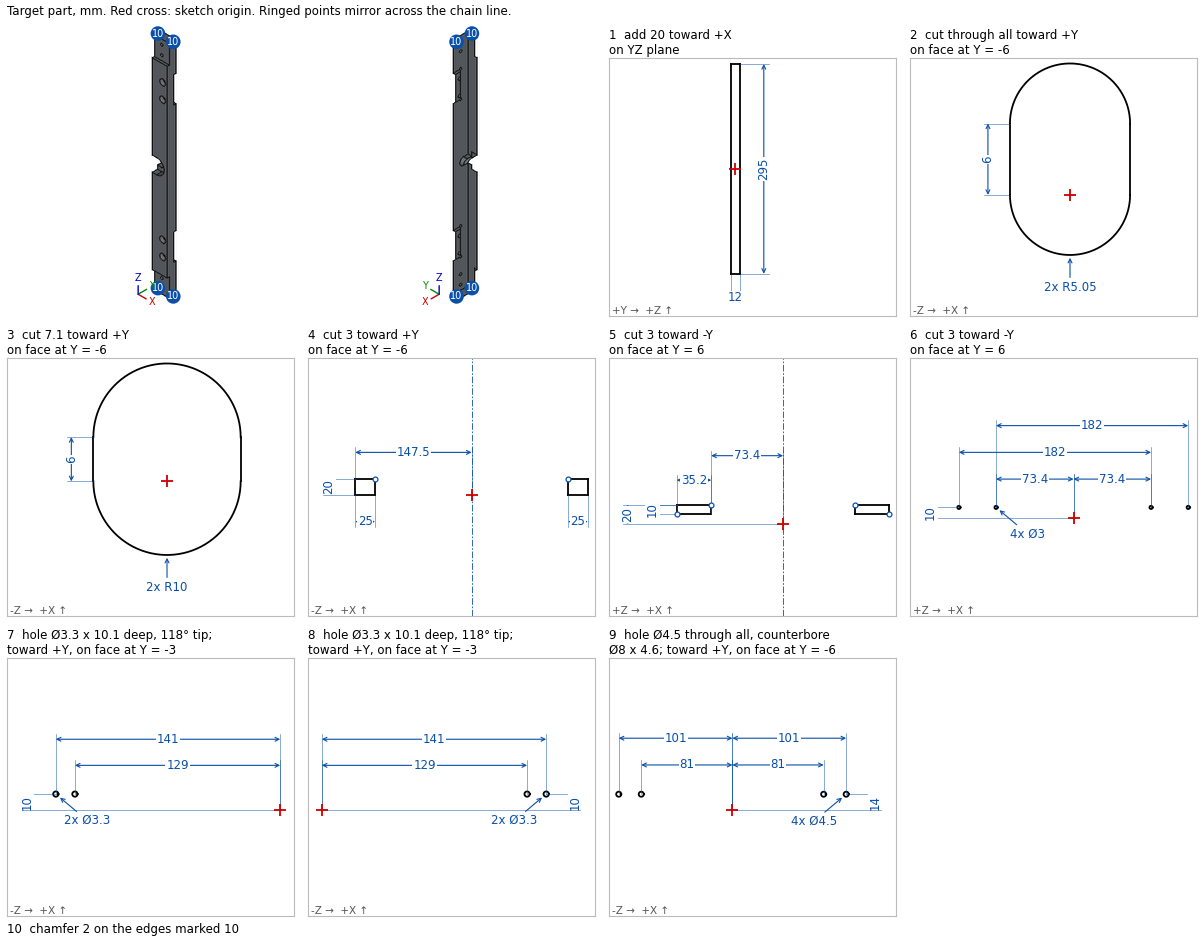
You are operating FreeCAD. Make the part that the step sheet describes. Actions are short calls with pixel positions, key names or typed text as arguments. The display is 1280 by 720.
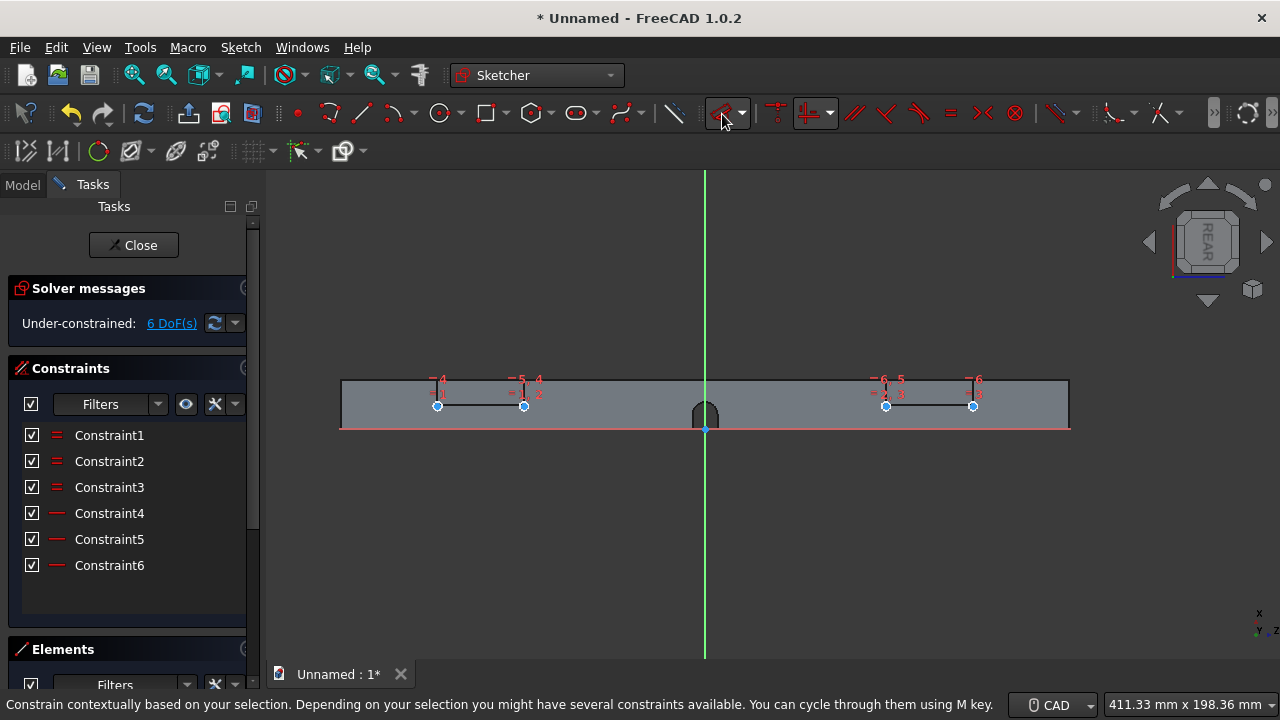
scroll(441, 403, up, 9)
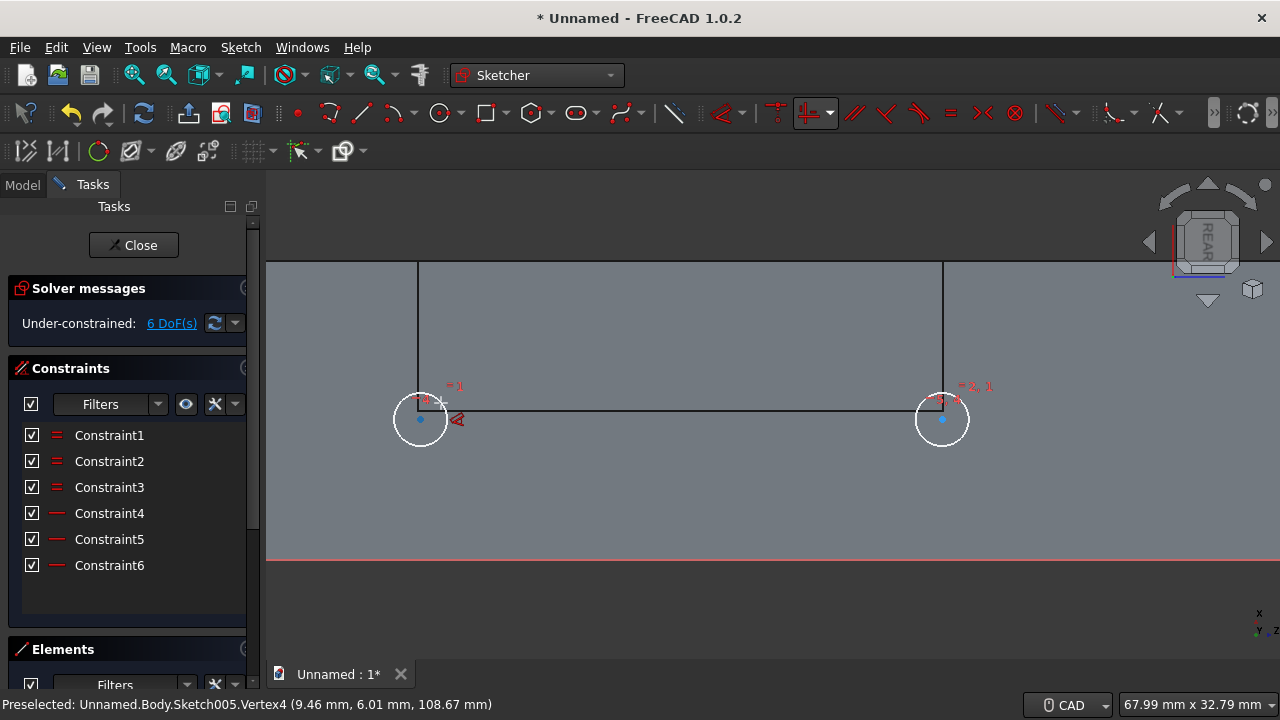
click(439, 401)
click(462, 378)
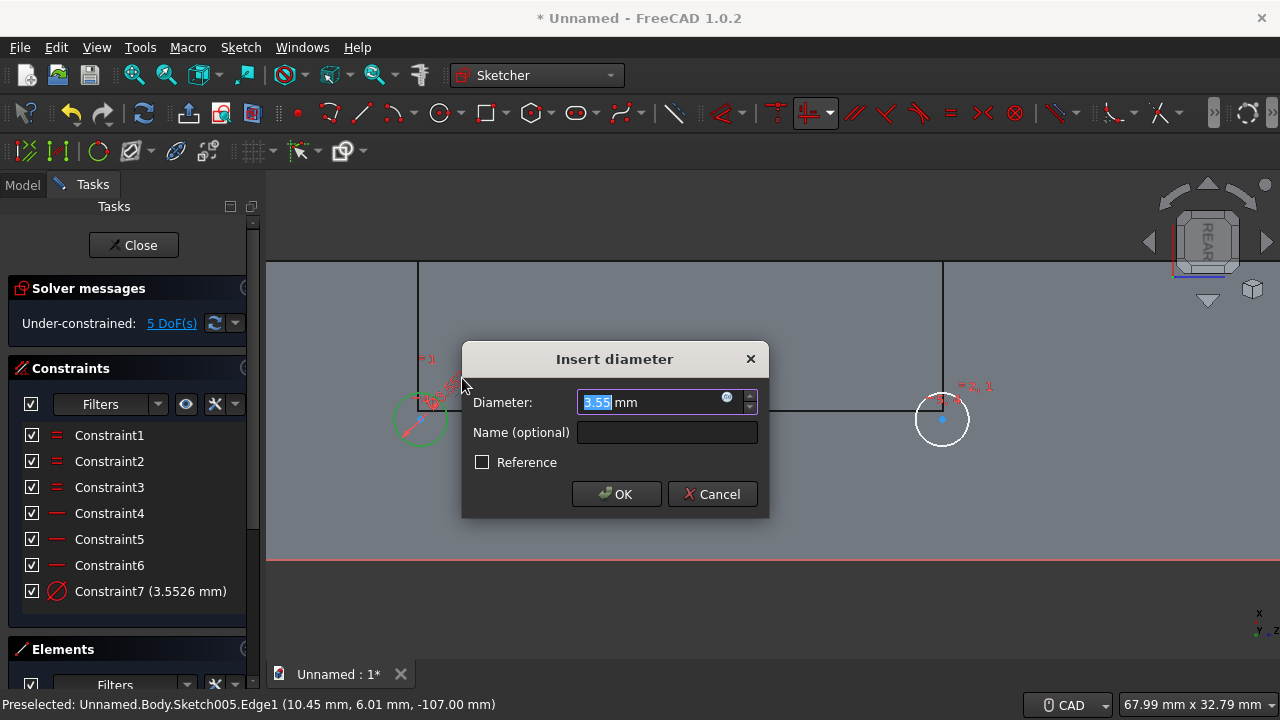
text(3)
key(Return)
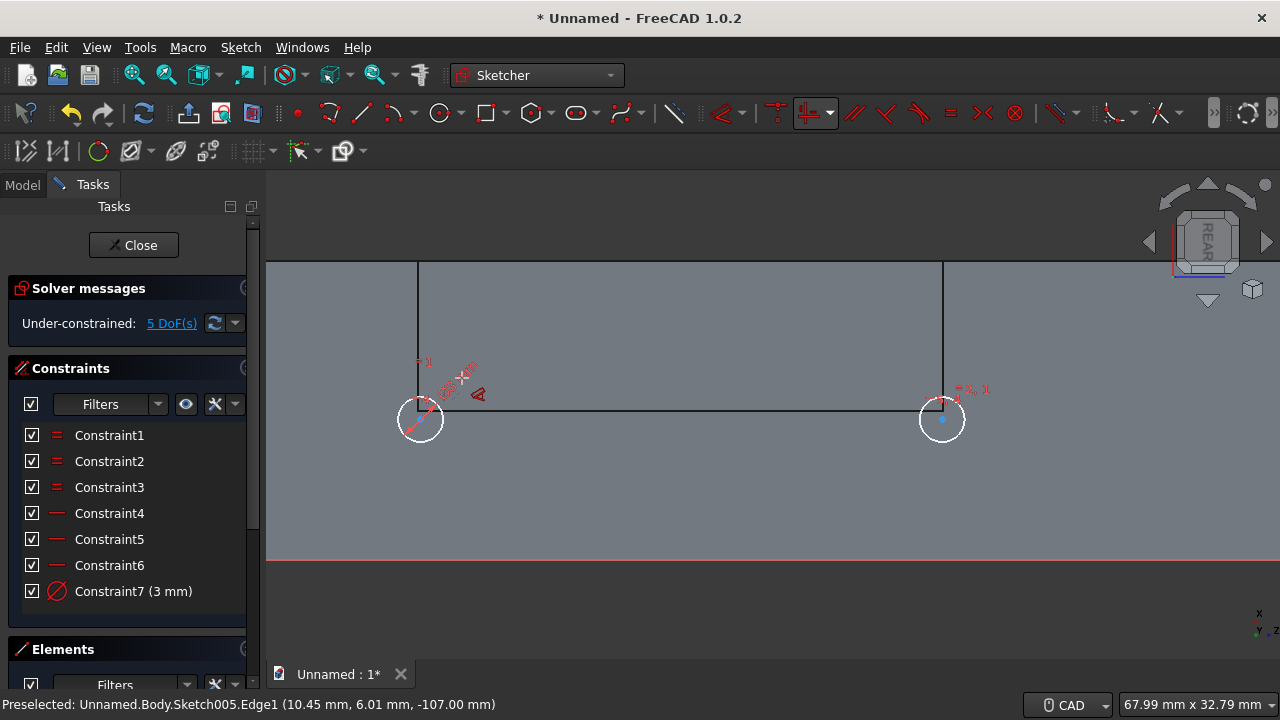
scroll(440, 403, down, 9)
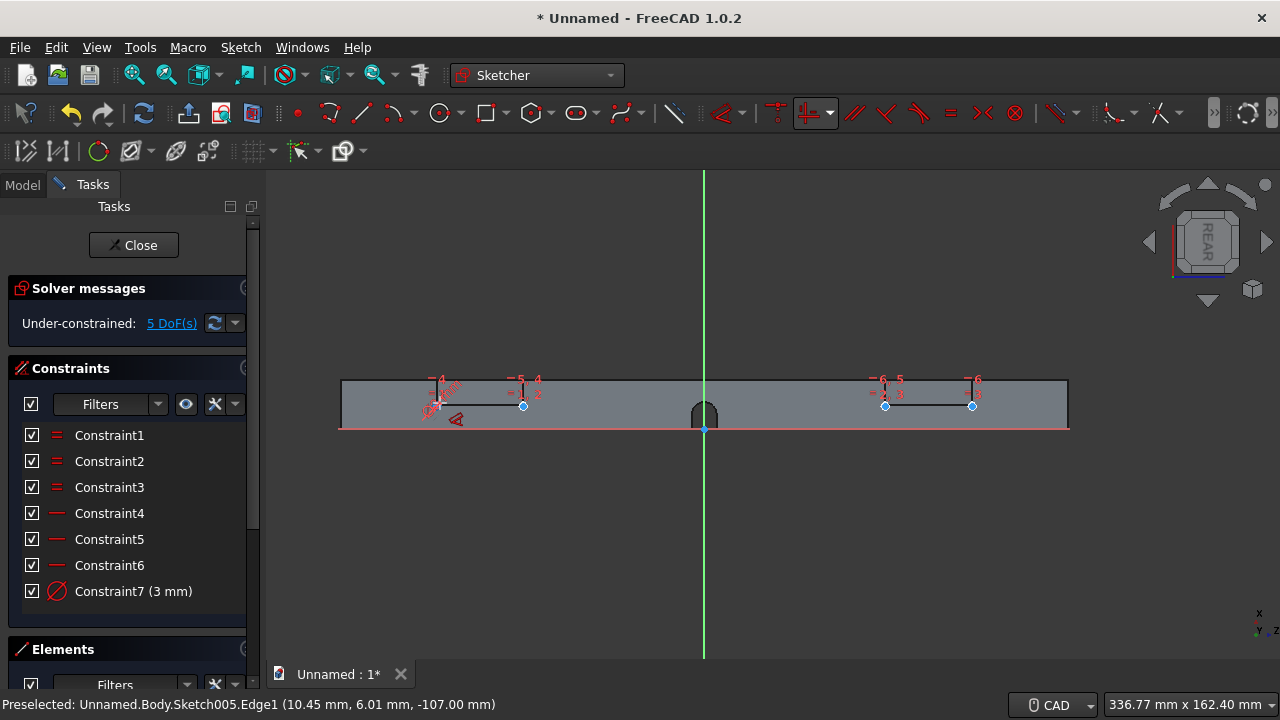
scroll(437, 406, up, 3)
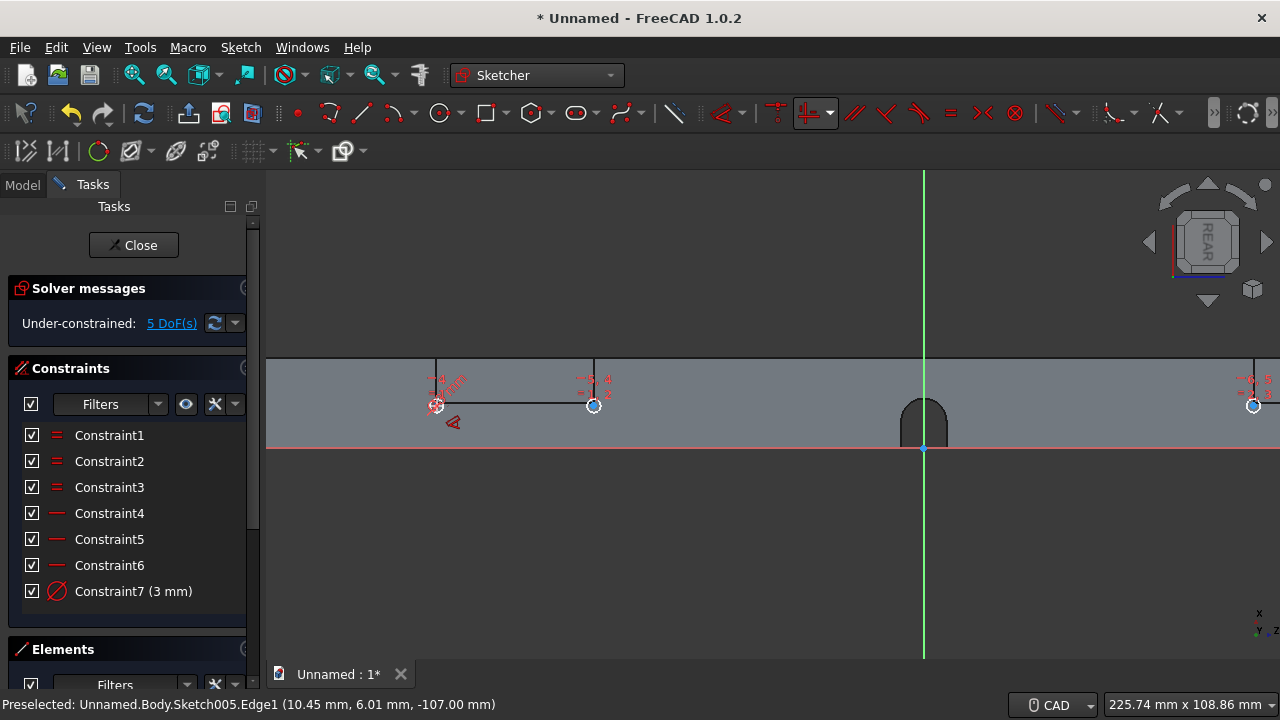
click(437, 406)
click(403, 427)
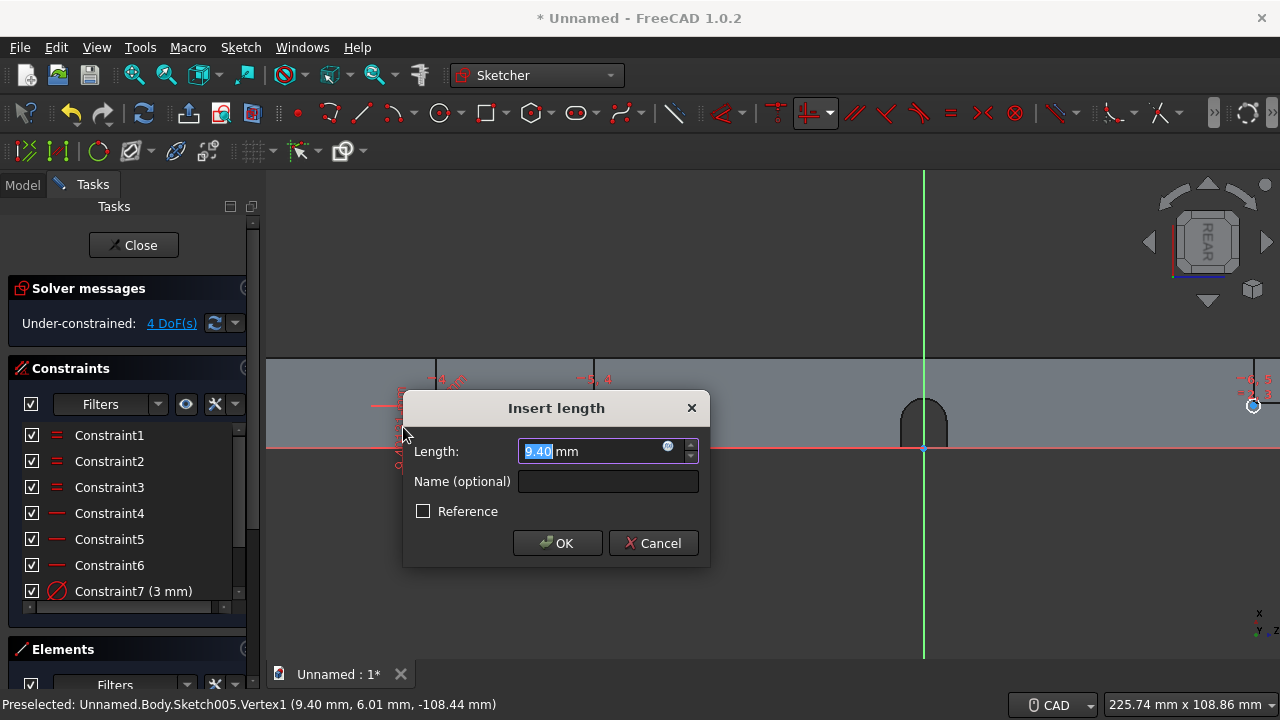
text(10)
key(Return)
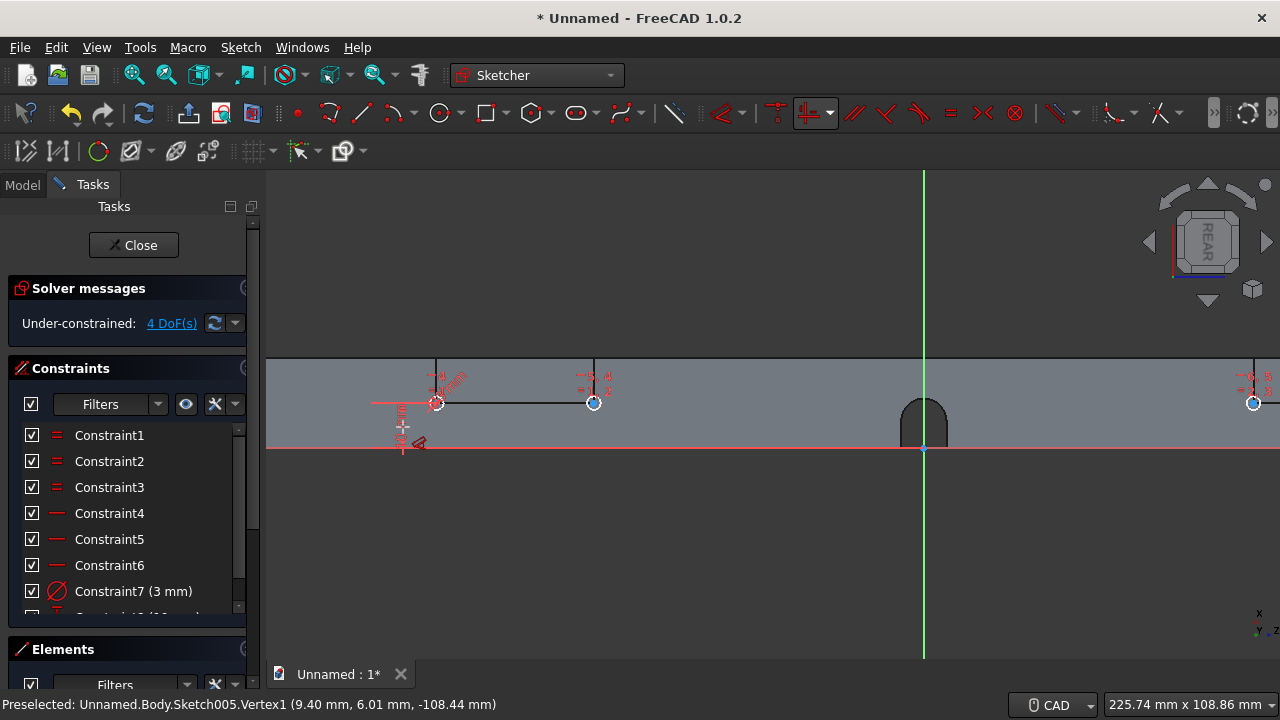
click(594, 403)
click(759, 482)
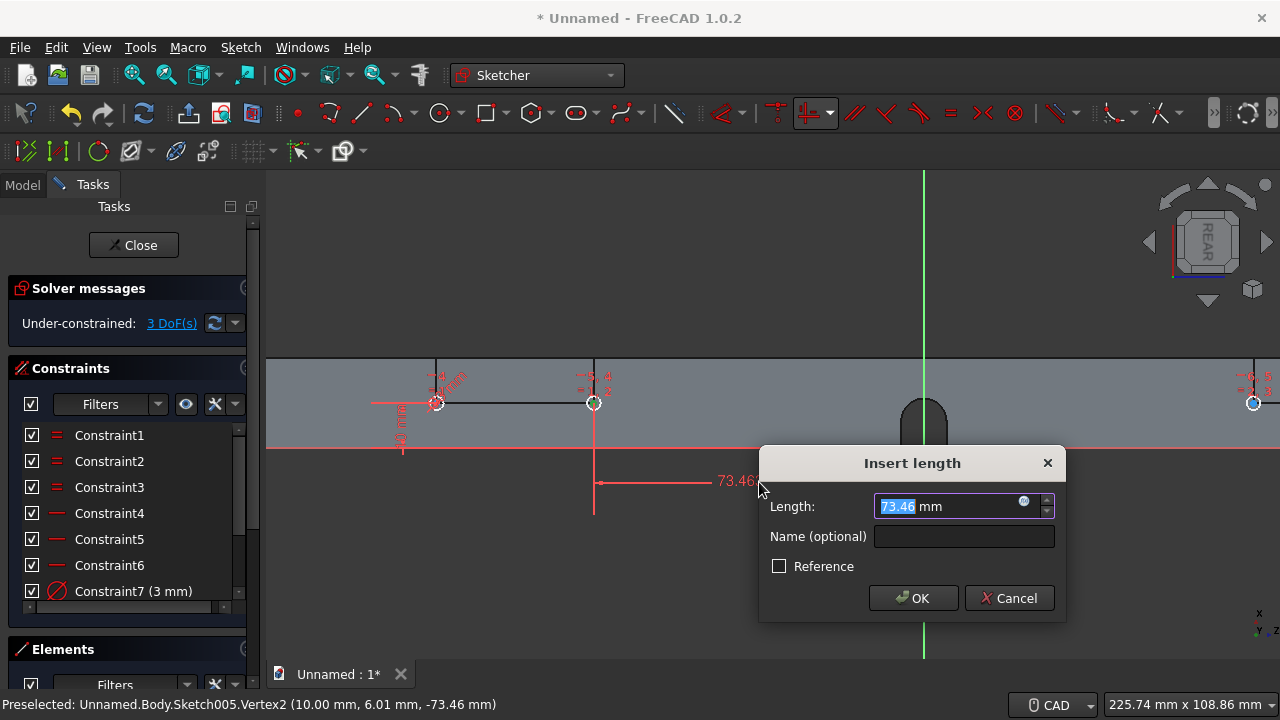
text(73.4)
key(Return)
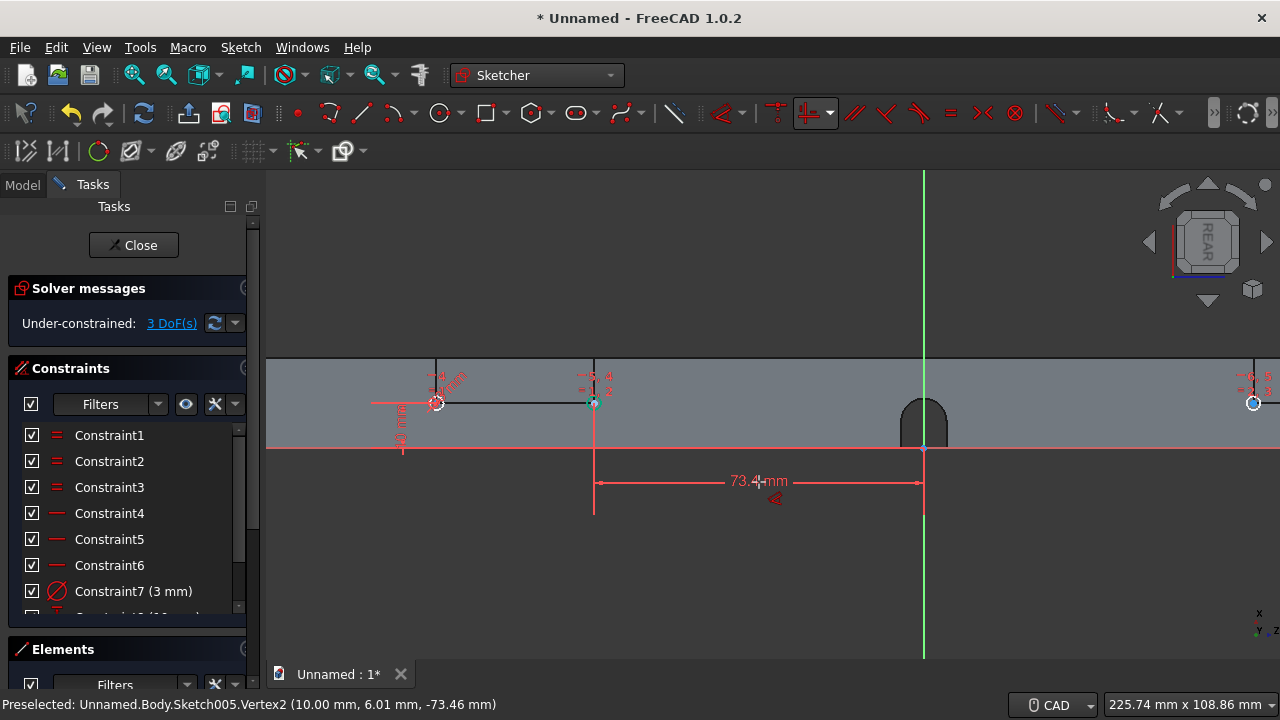
scroll(438, 405, down, 3)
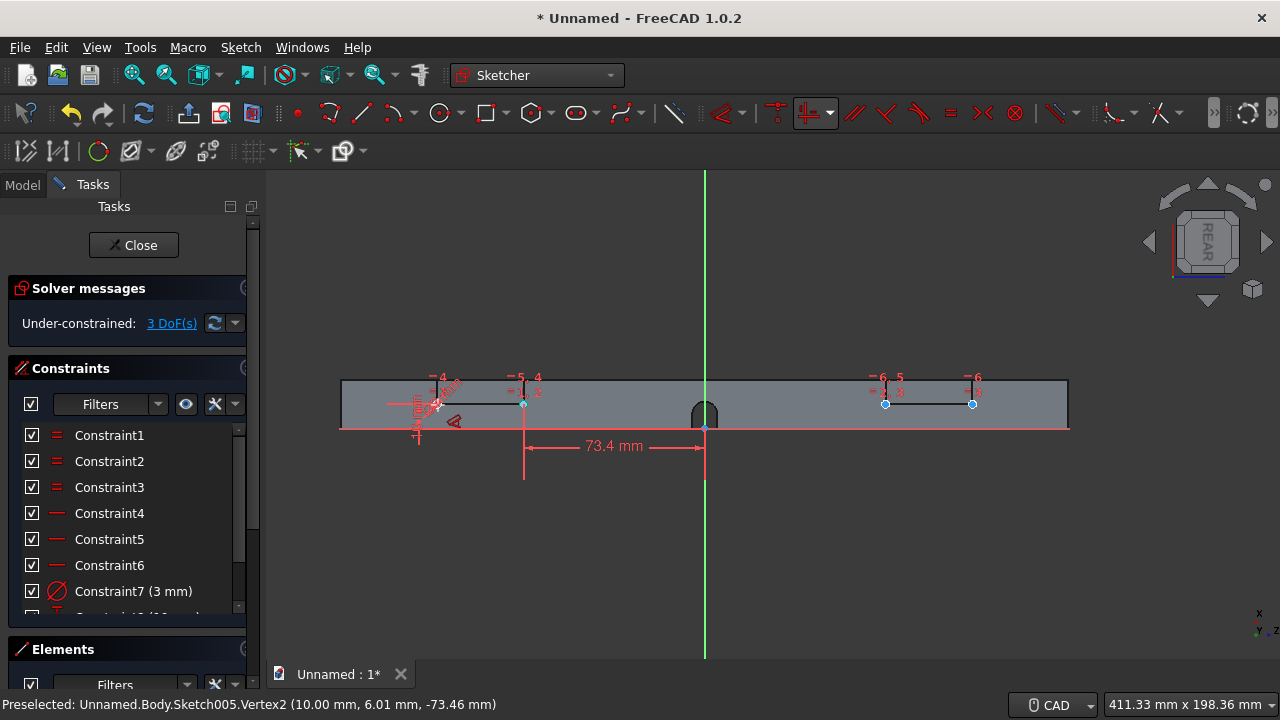
click(886, 404)
click(795, 463)